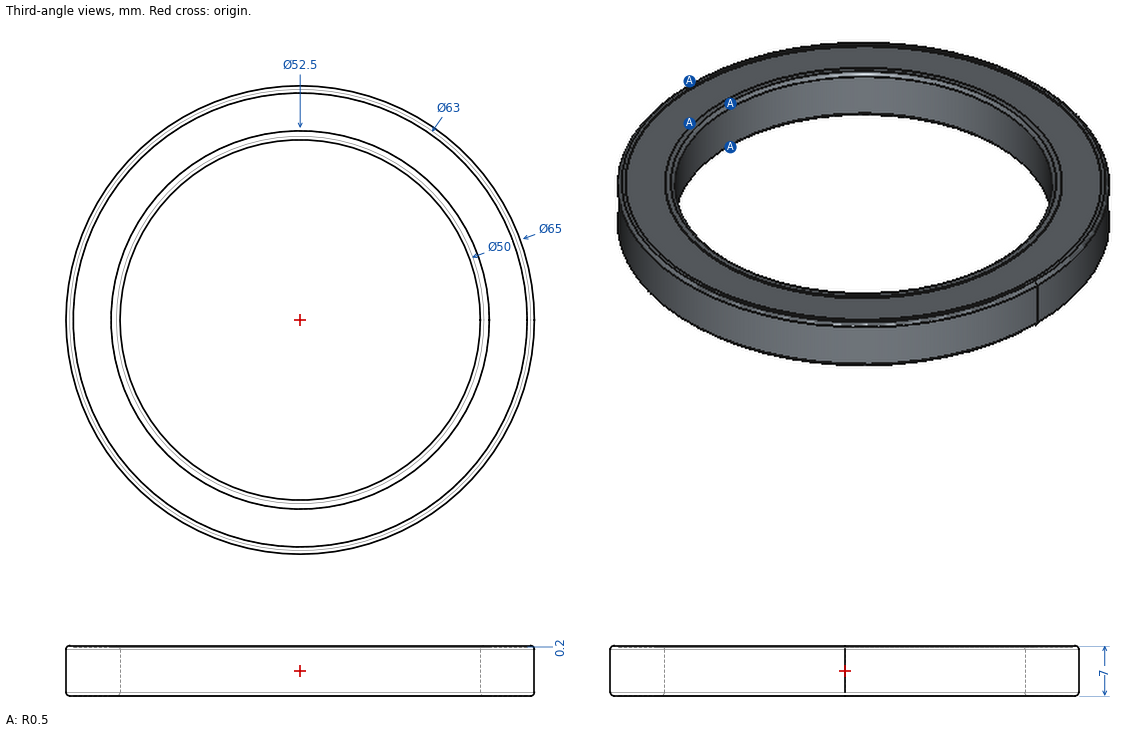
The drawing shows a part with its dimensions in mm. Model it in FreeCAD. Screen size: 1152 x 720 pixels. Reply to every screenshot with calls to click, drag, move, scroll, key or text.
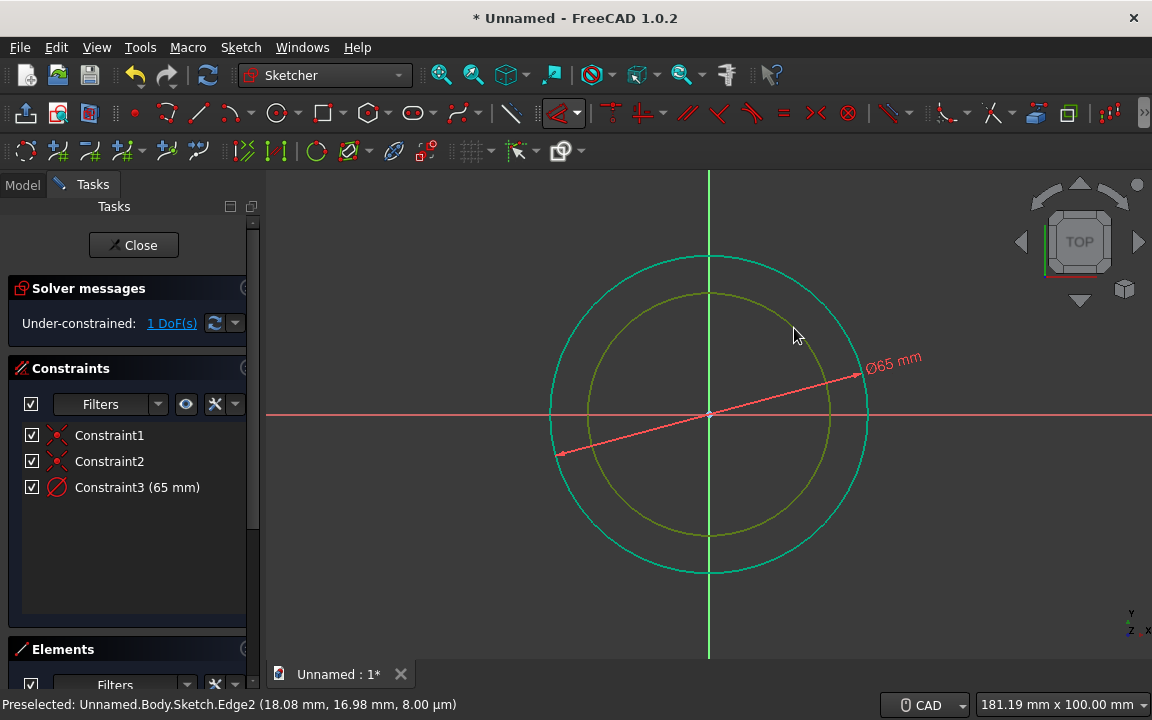
key(k)
key(o)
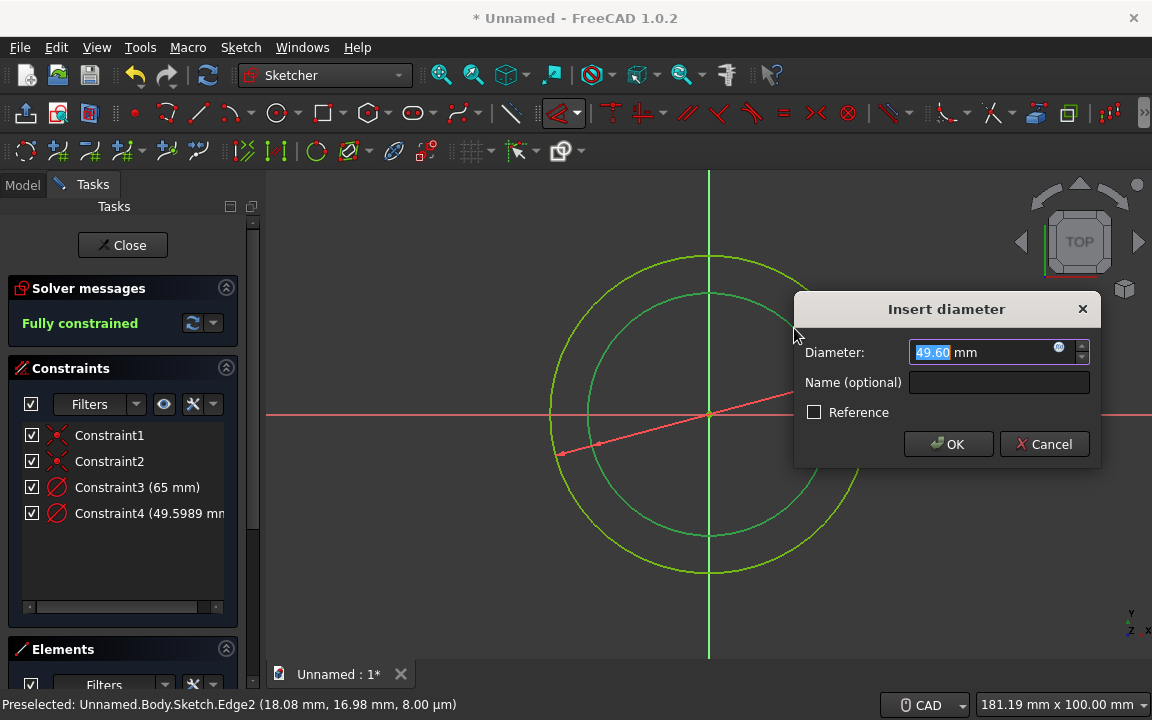
text(50)
key(Return)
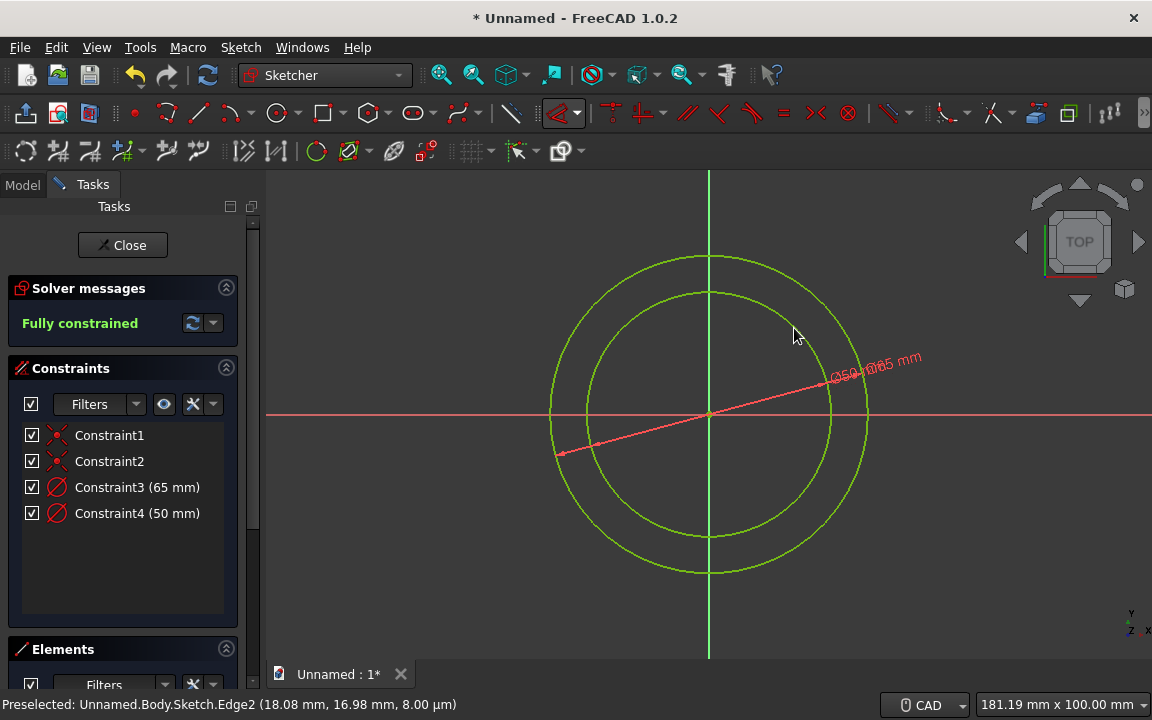
click(123, 245)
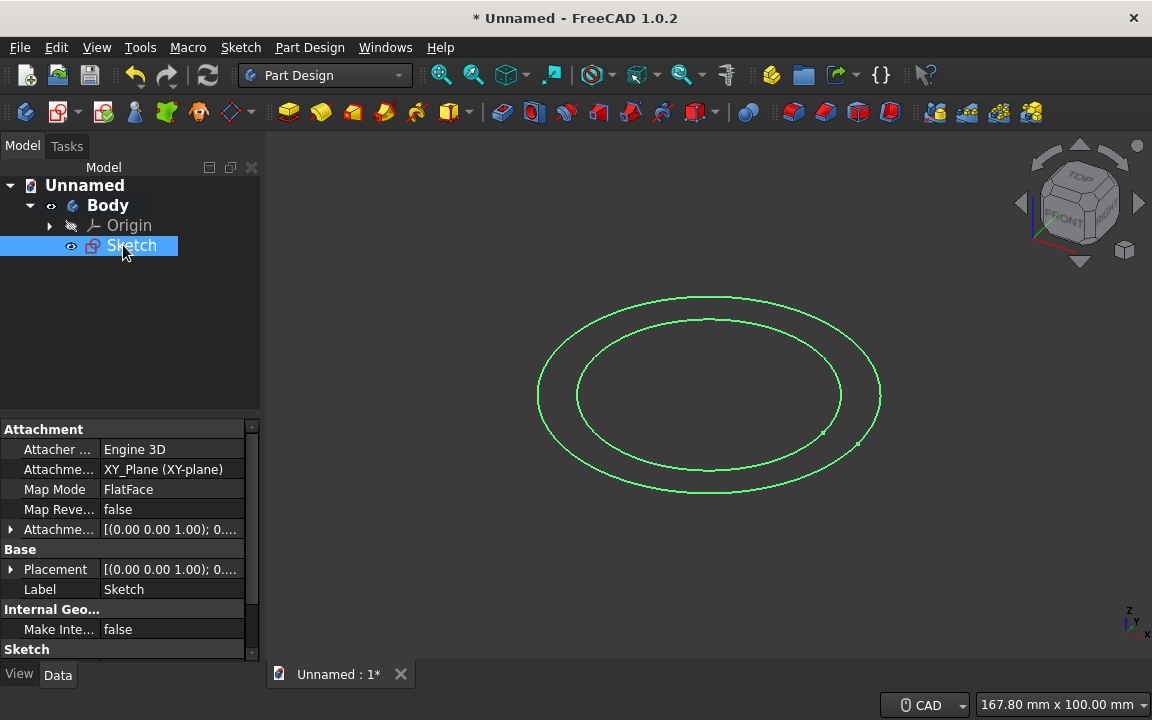
click(290, 112)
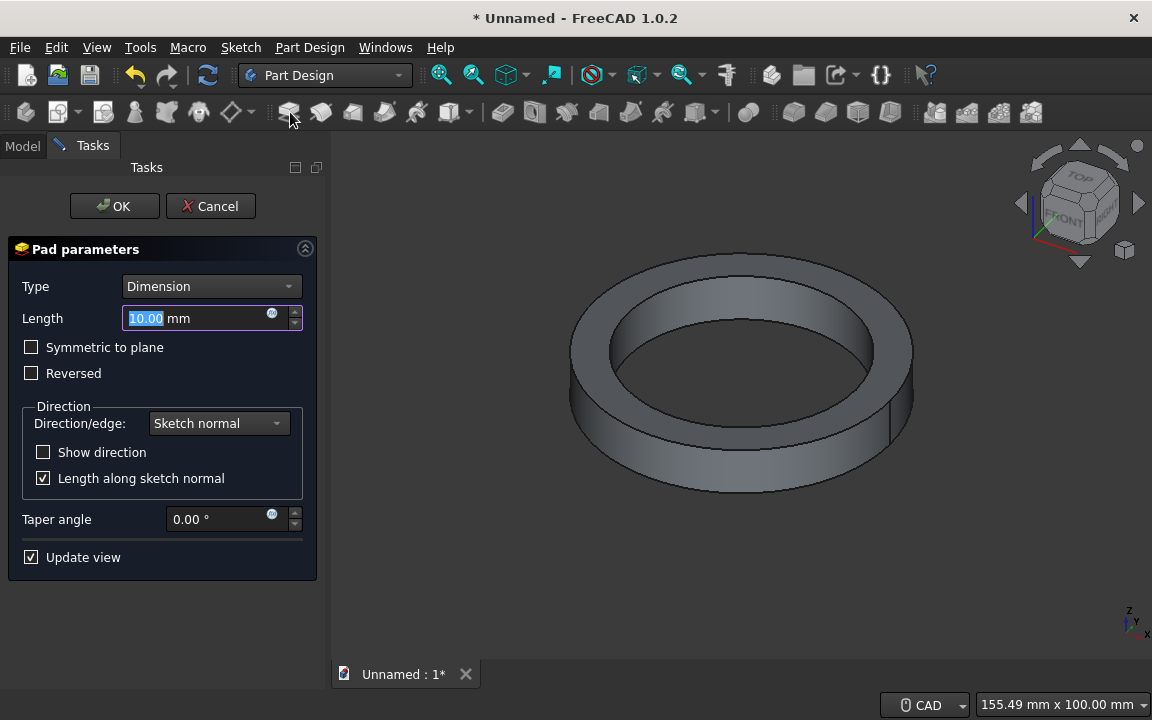
text(7)
key(Tab)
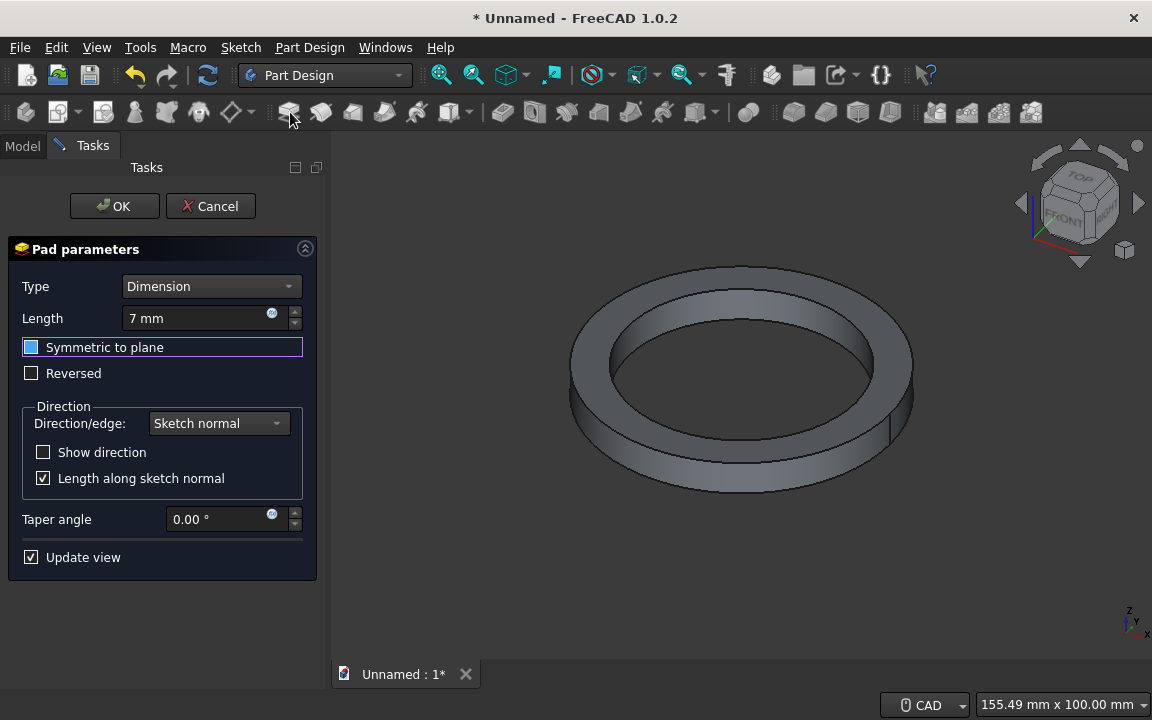
click(30, 347)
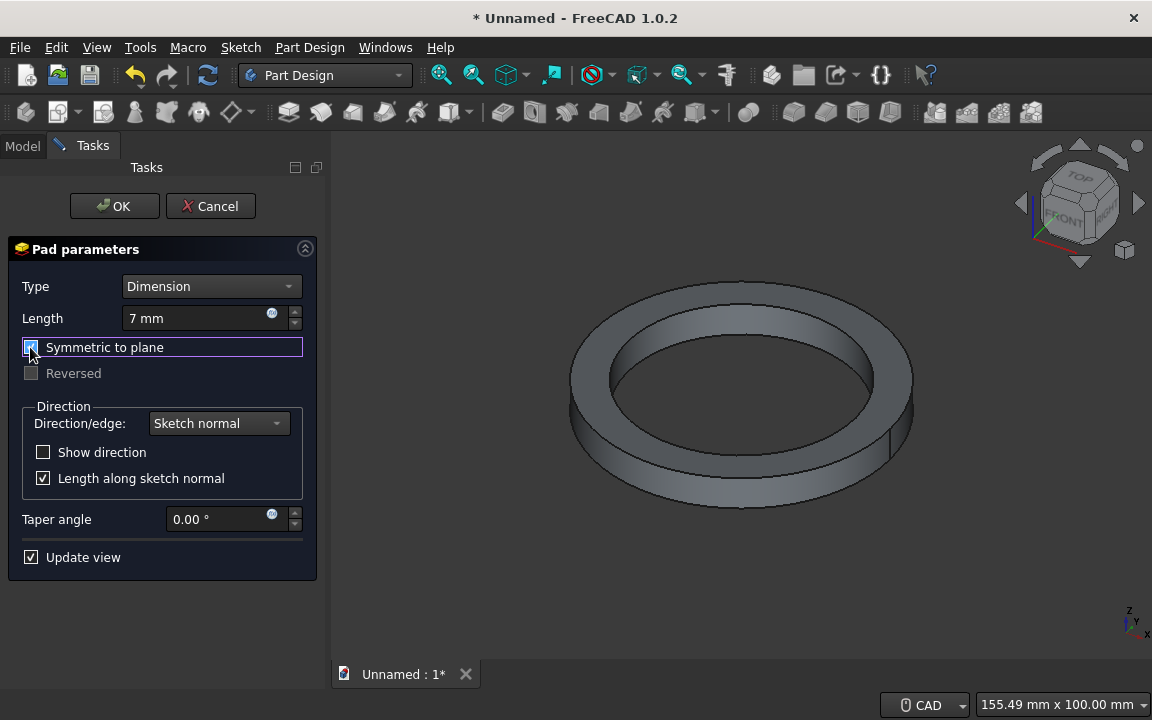
click(115, 206)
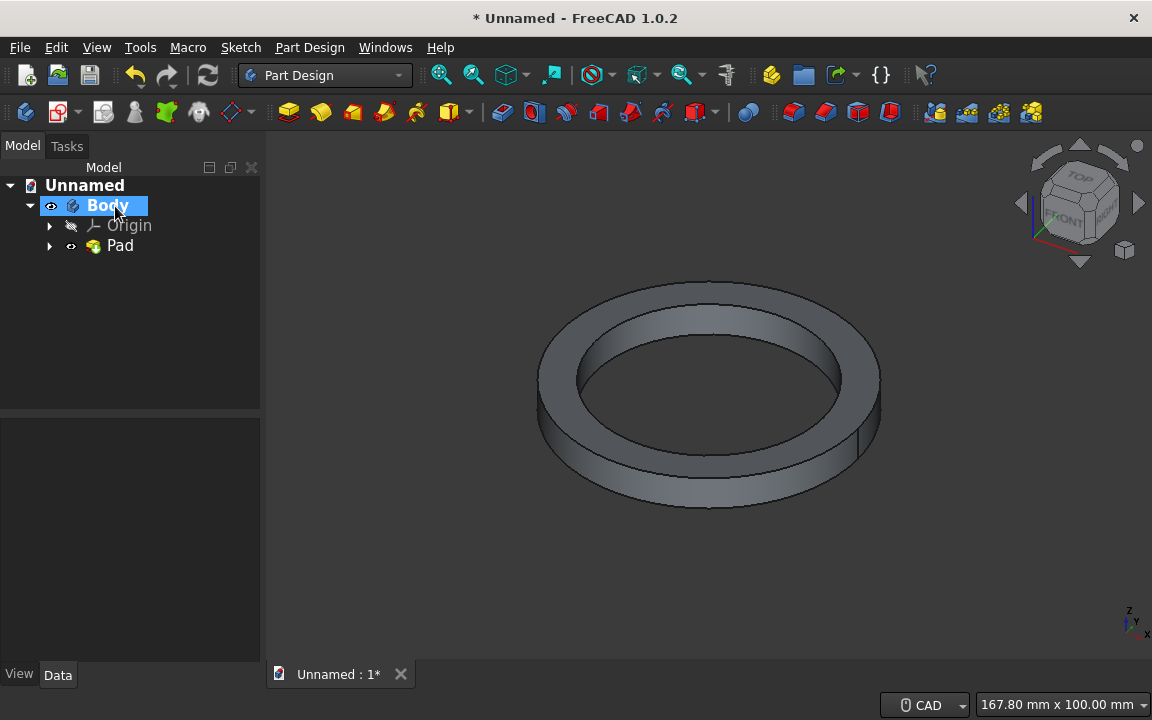
click(812, 445)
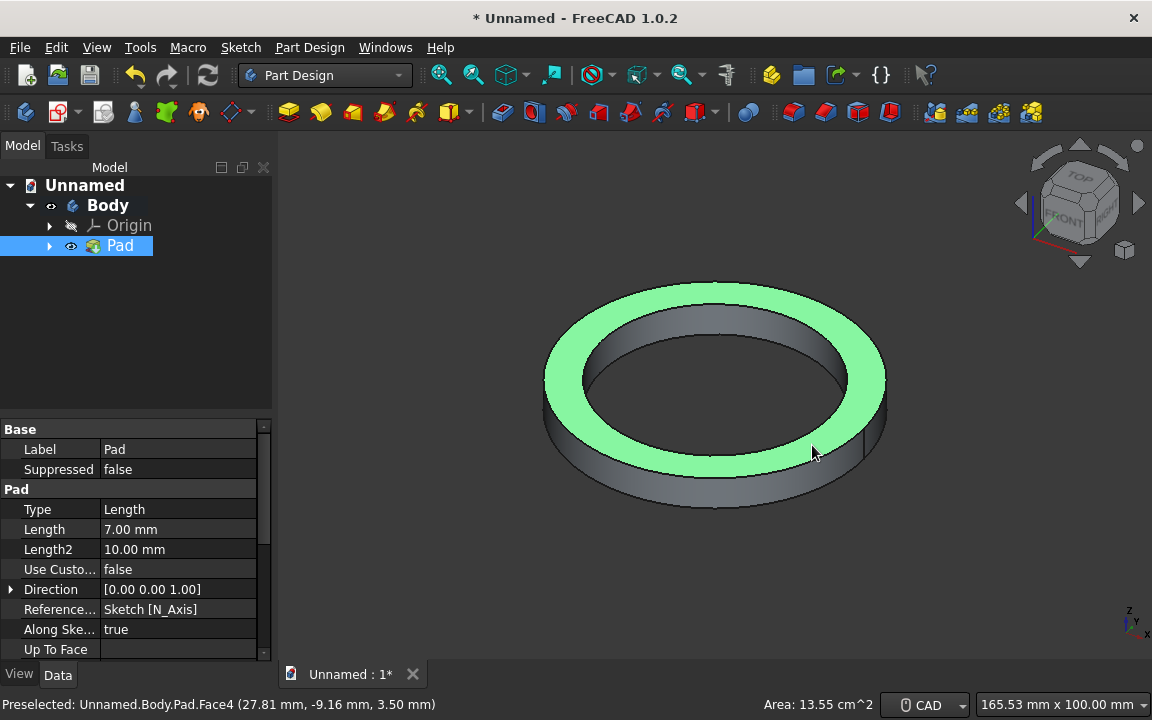
click(58, 112)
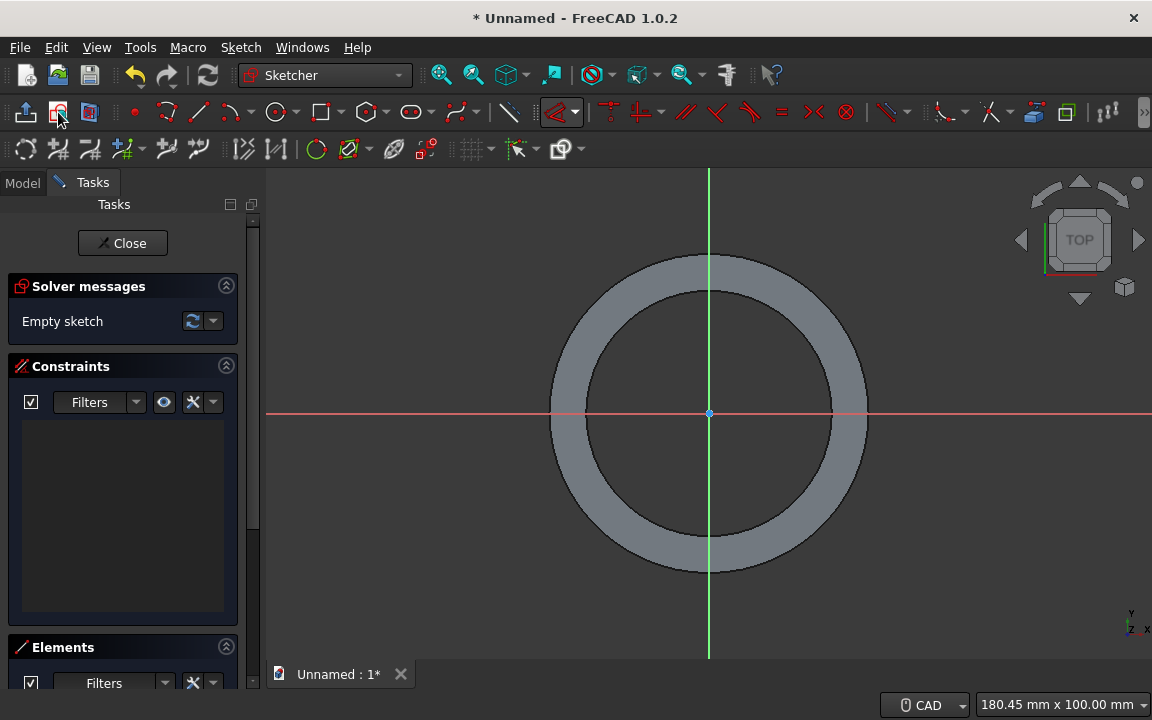
click(276, 112)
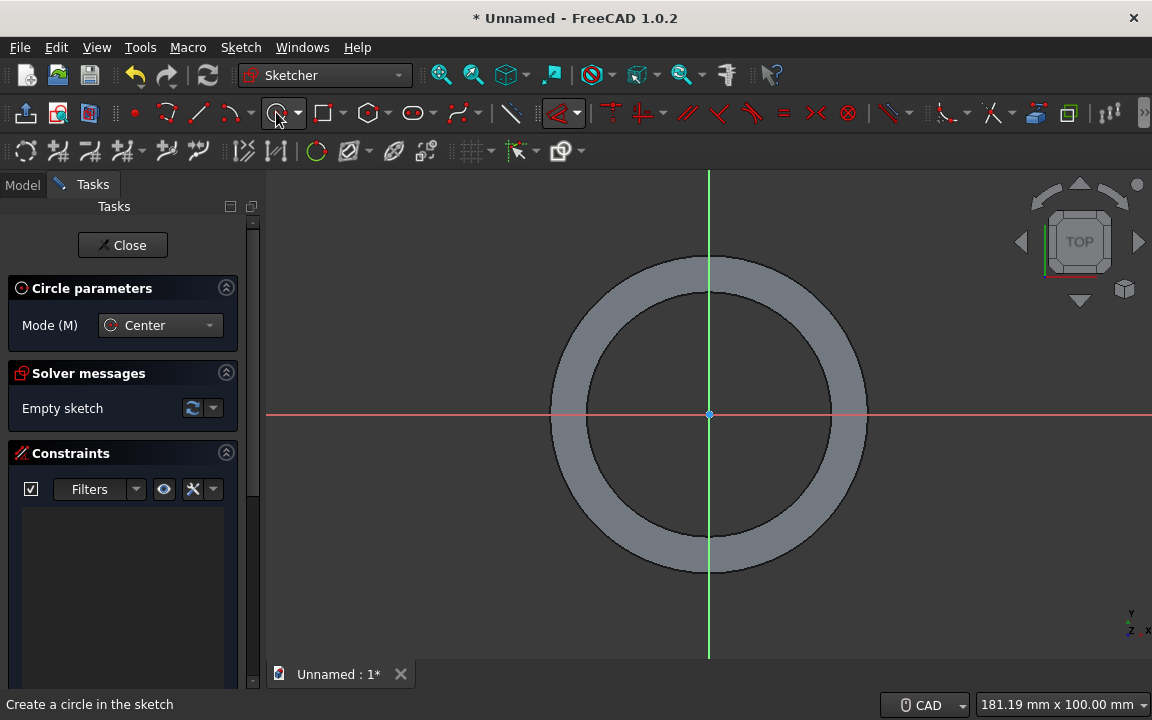
click(709, 414)
click(818, 306)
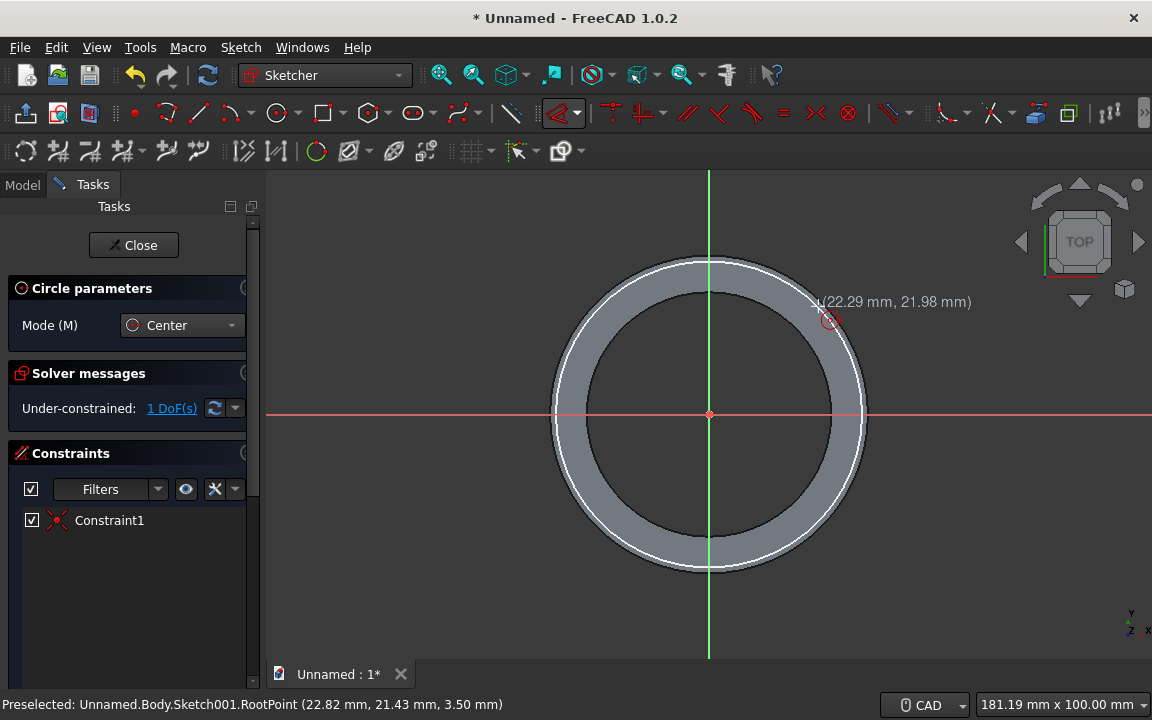
click(709, 414)
click(800, 324)
key(Escape)